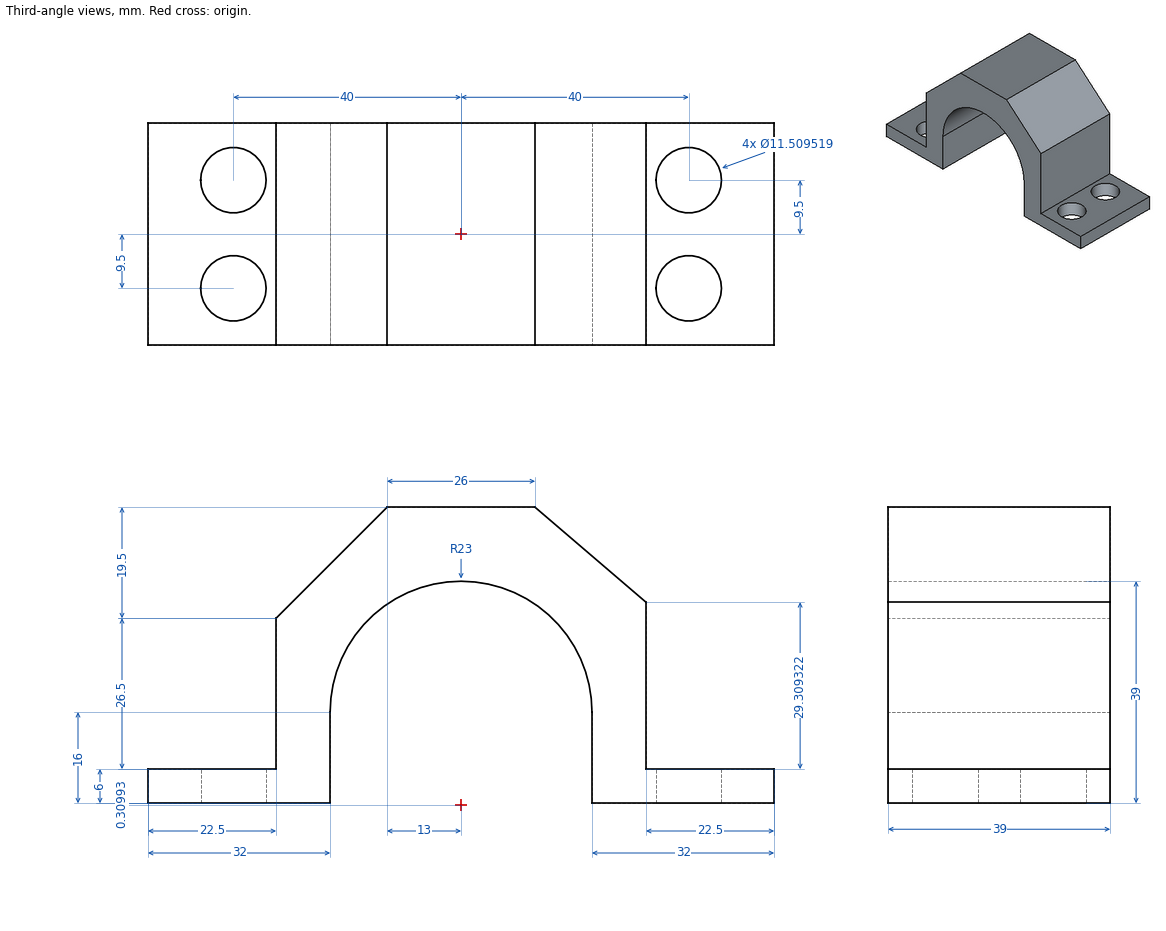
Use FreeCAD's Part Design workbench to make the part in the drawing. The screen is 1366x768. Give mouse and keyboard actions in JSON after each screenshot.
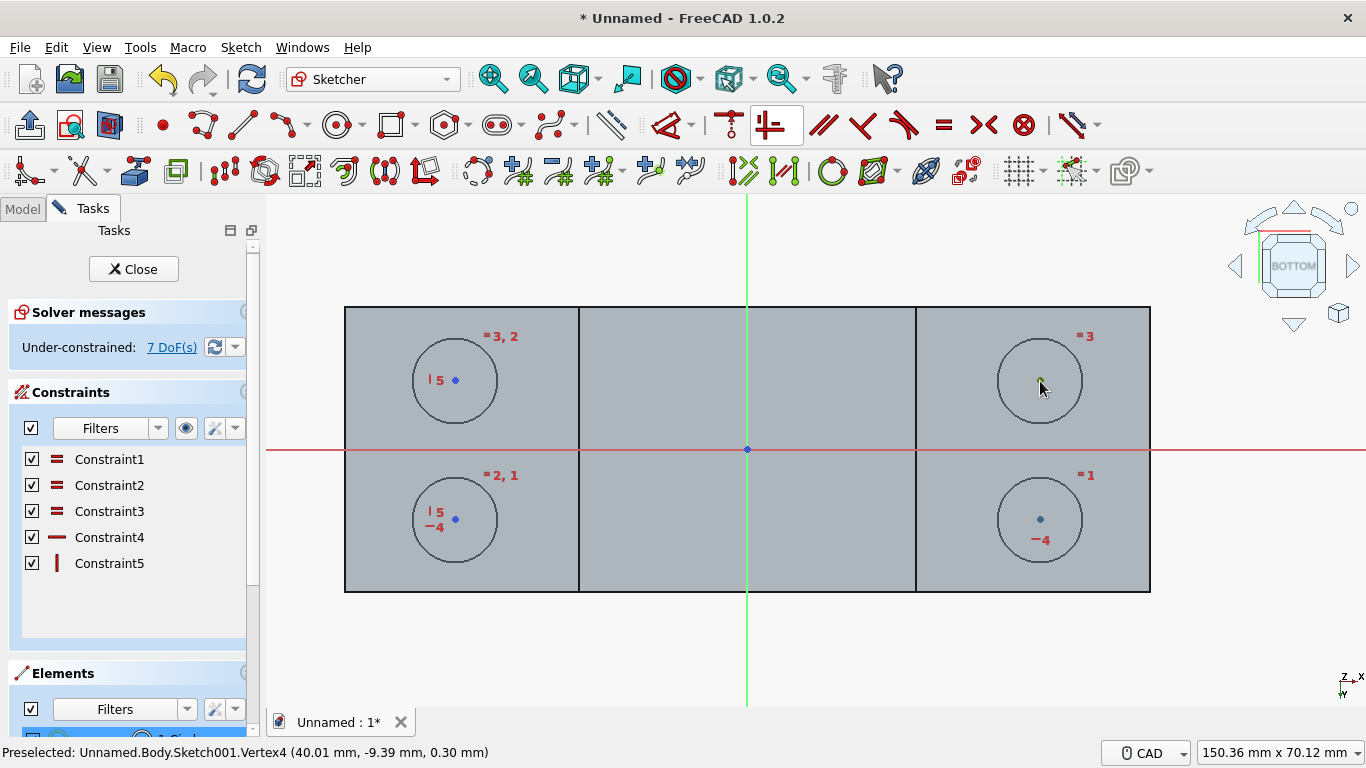
{"action": "key", "text": "v"}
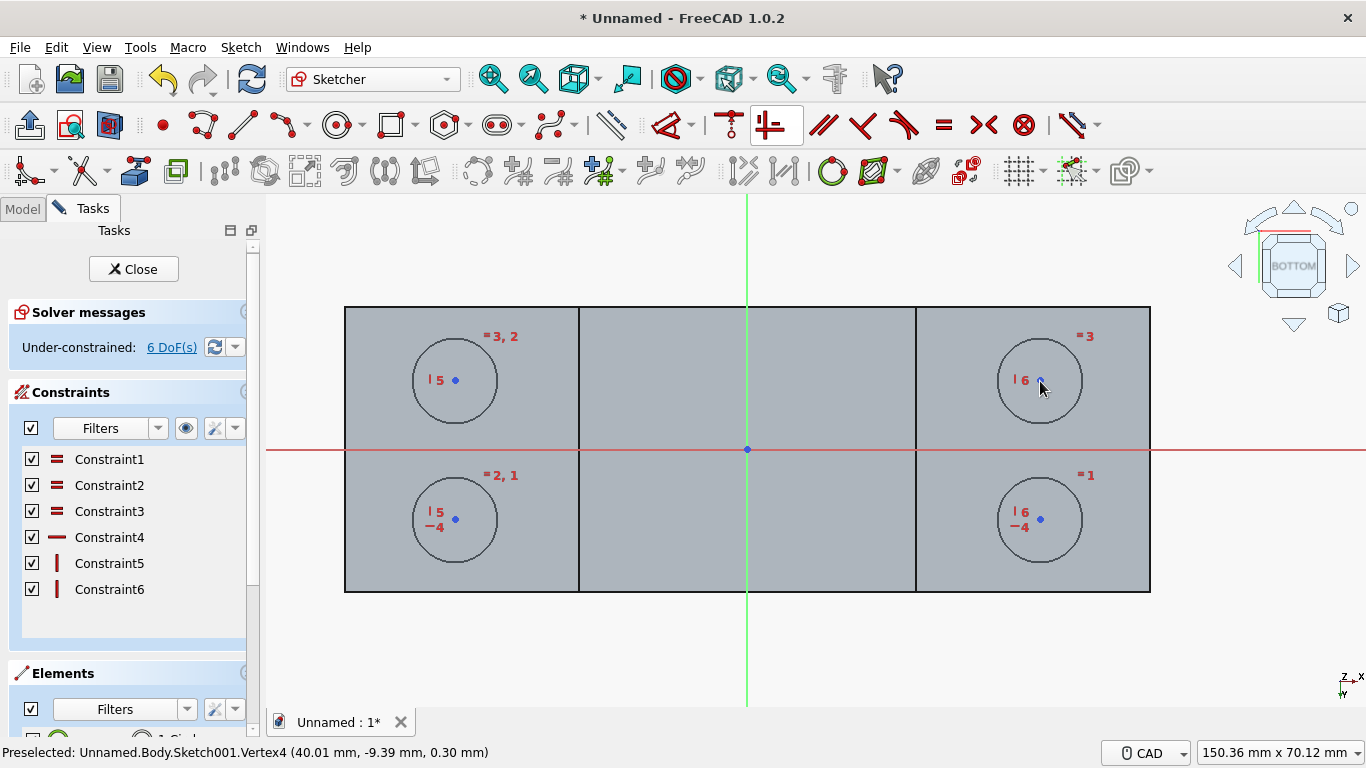
{"action": "left_click", "coordinate": [455, 381]}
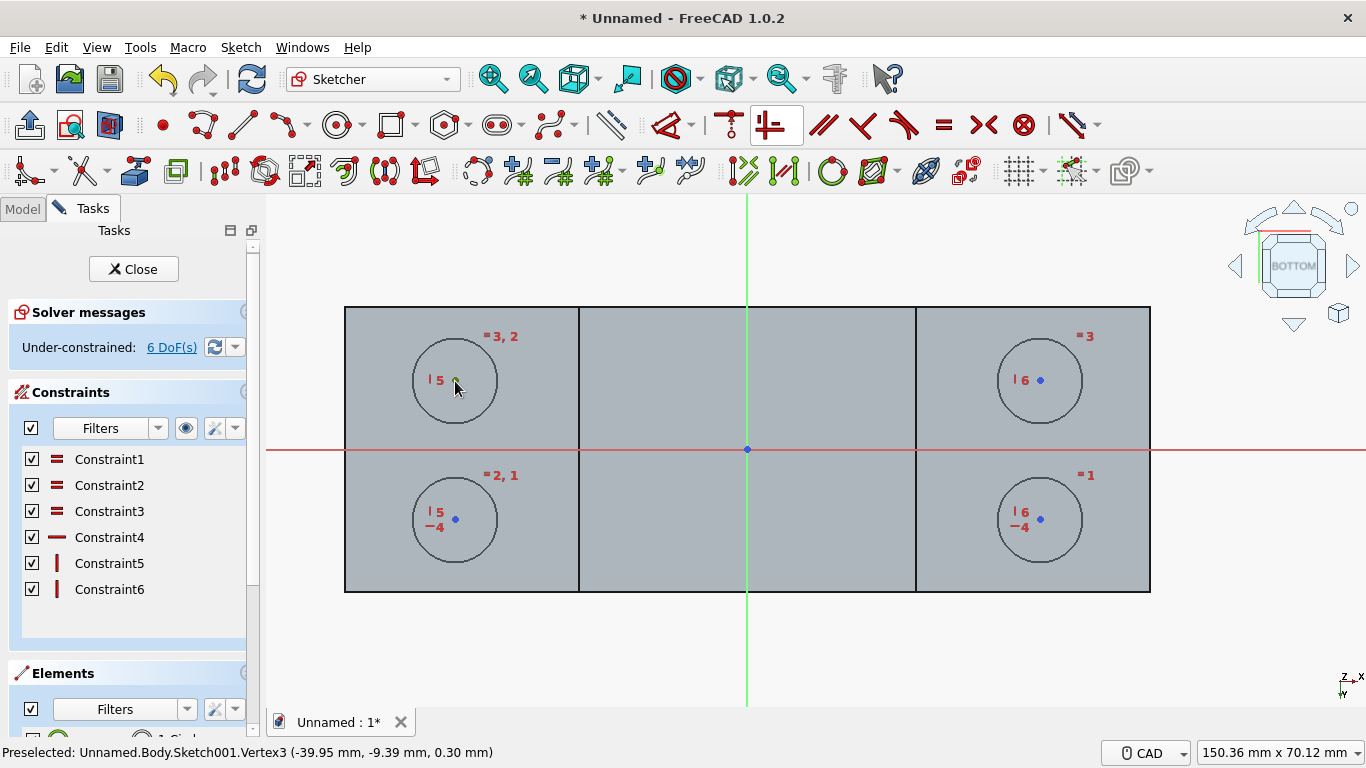
{"action": "left_click", "coordinate": [1040, 381]}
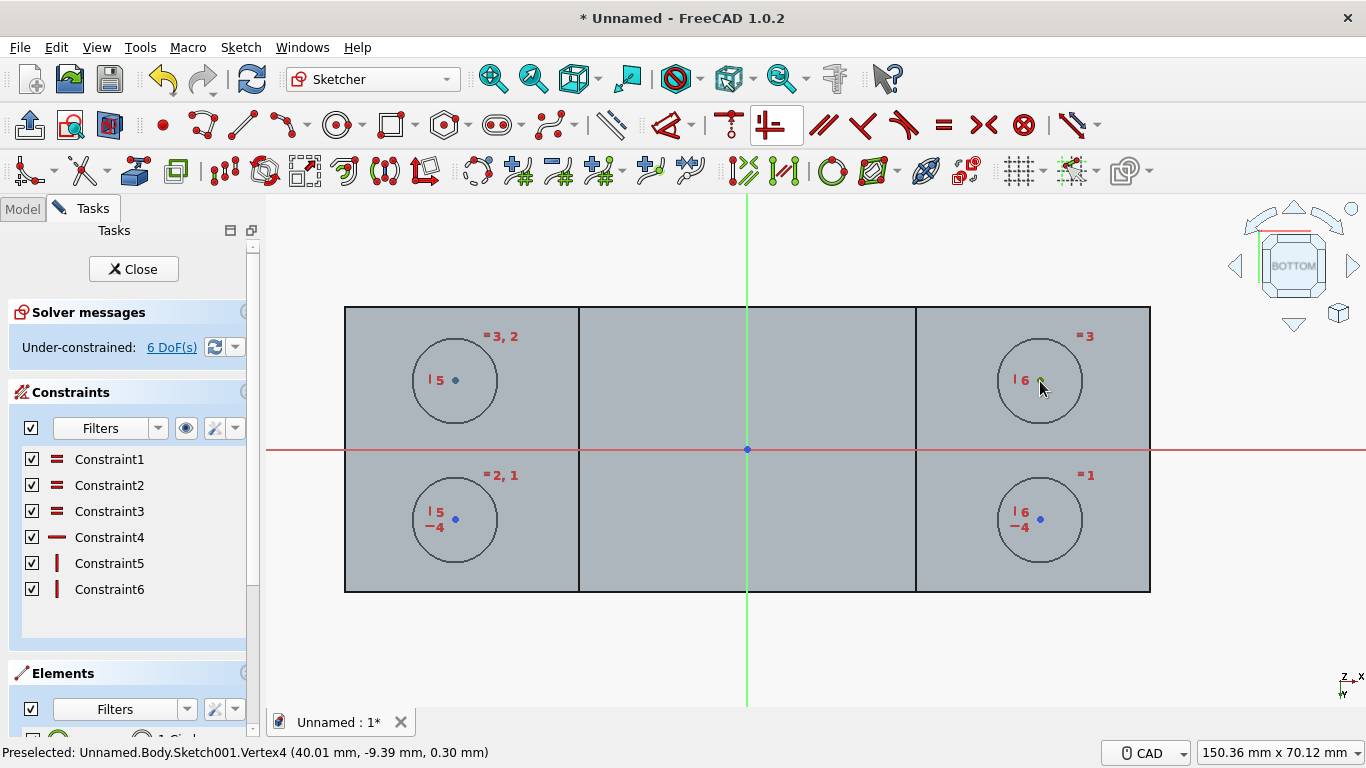
{"action": "key", "text": "h"}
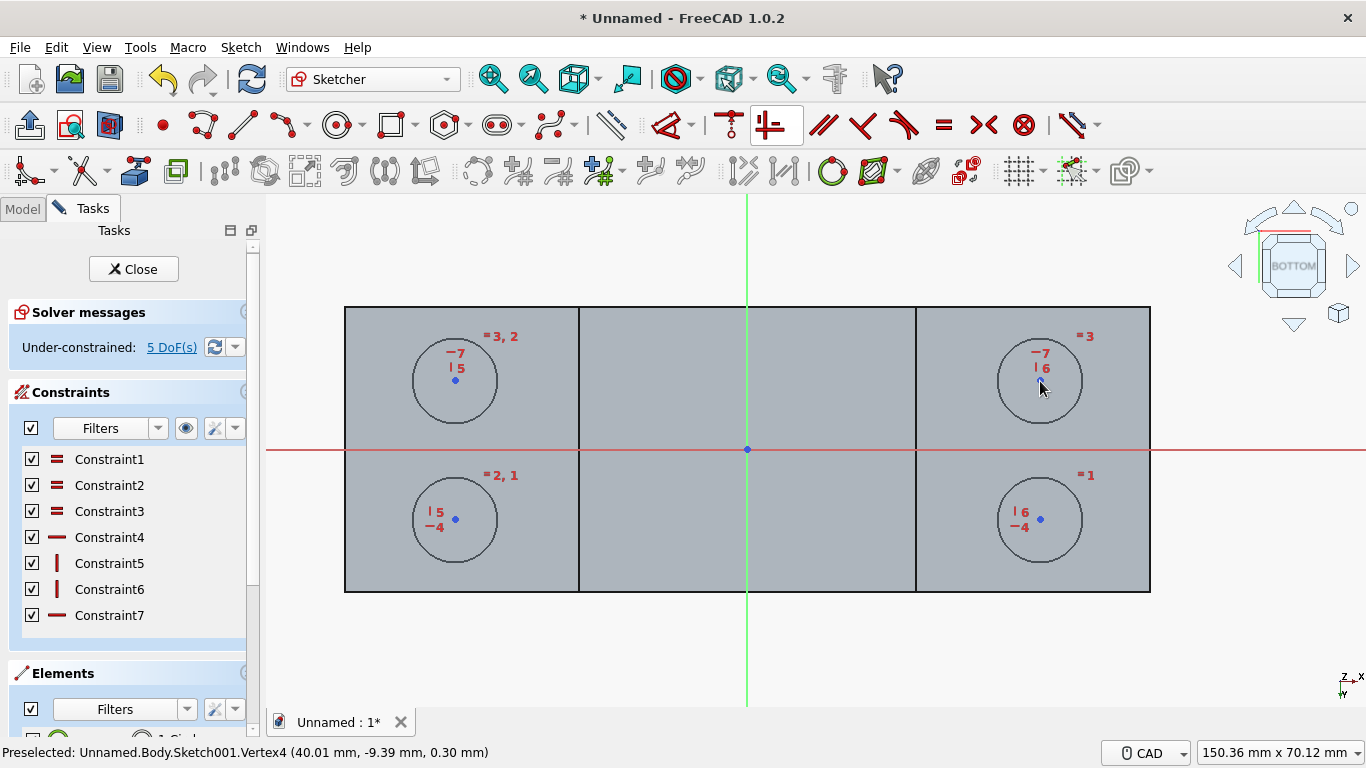
{"action": "left_click", "coordinate": [666, 126]}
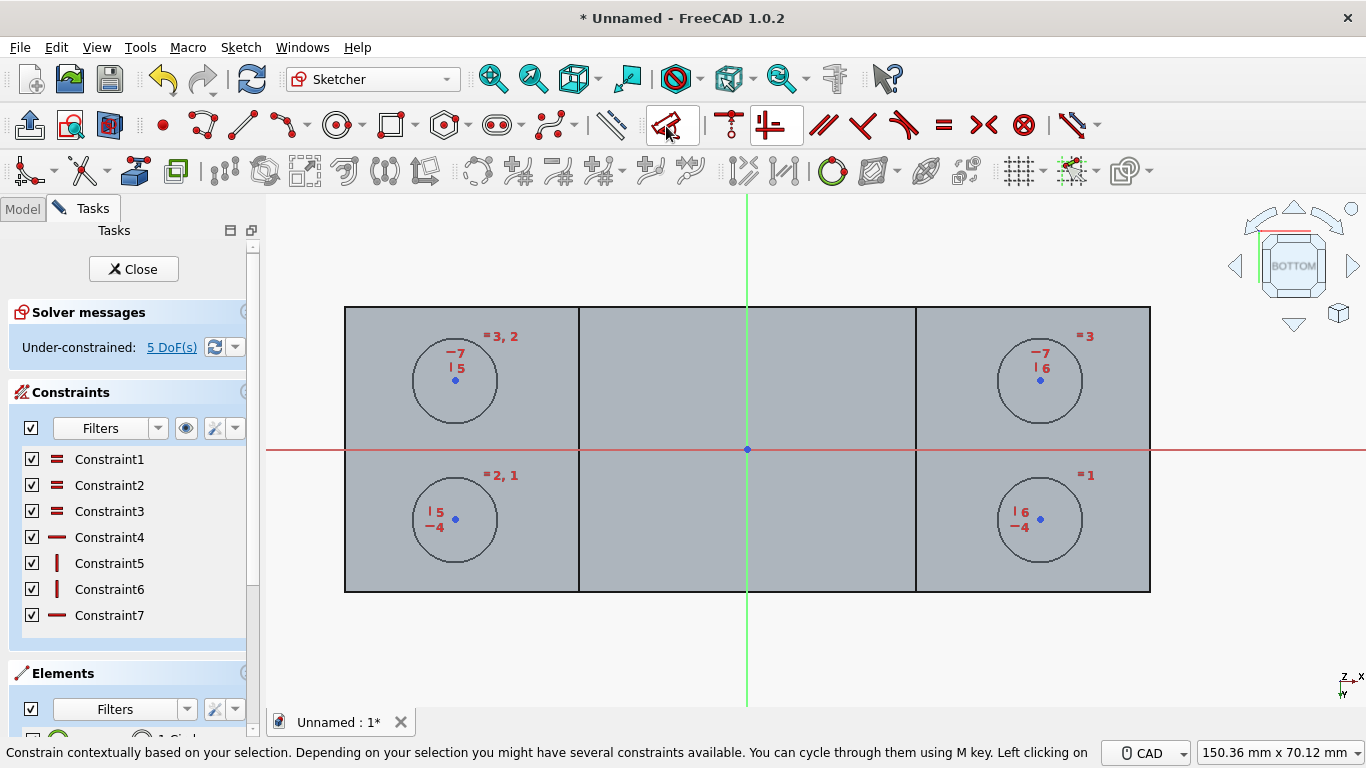
{"action": "left_click", "coordinate": [1070, 490]}
{"action": "left_click", "coordinate": [1093, 467]}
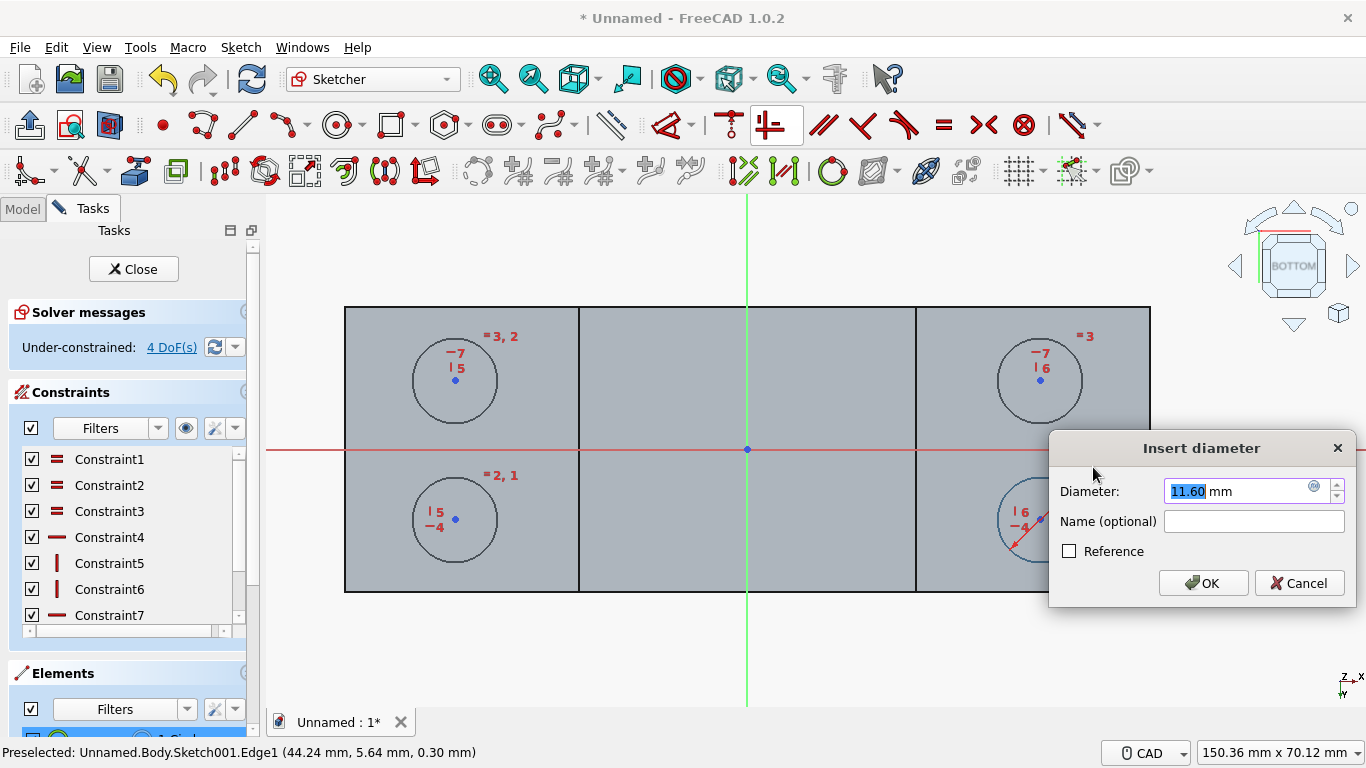
{"action": "type", "text": "11.509519"}
{"action": "key", "text": "Return"}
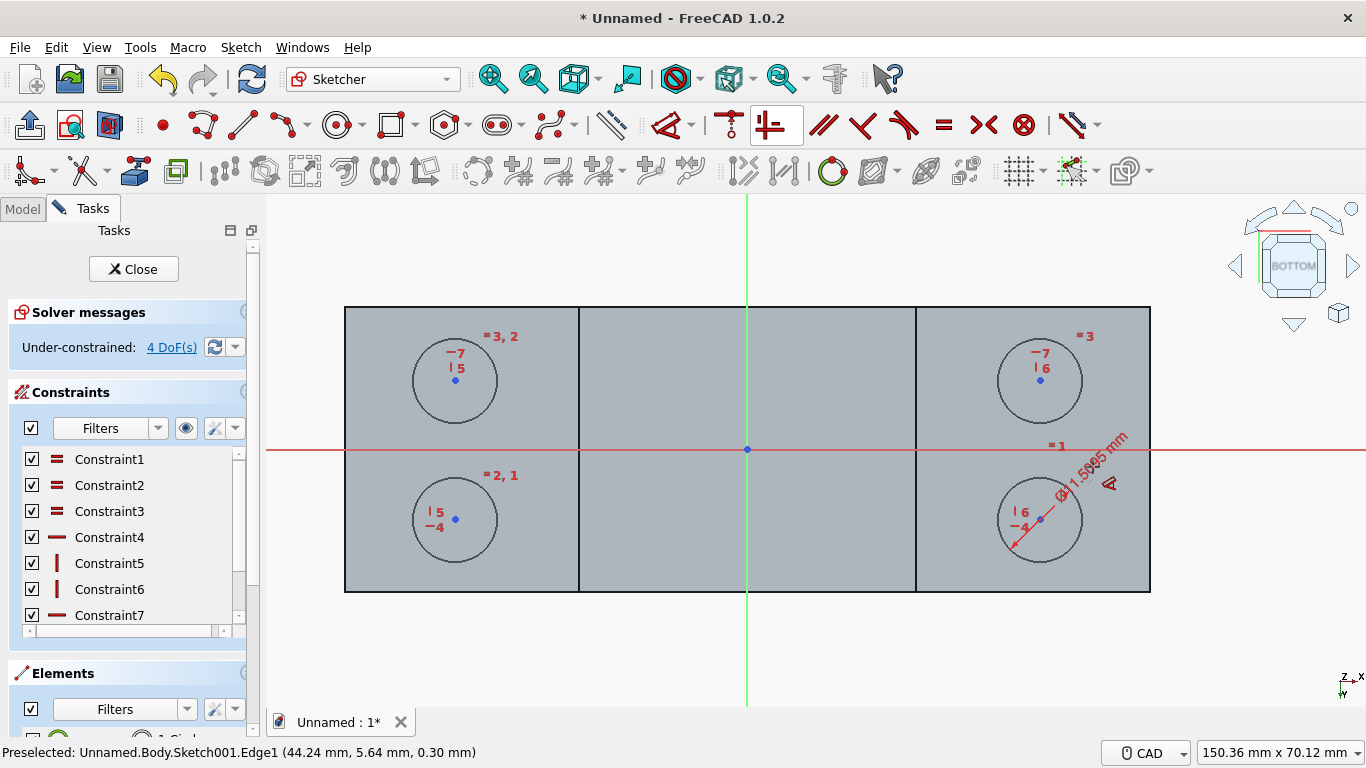
{"action": "left_click", "coordinate": [1040, 520]}
{"action": "left_click", "coordinate": [894, 554]}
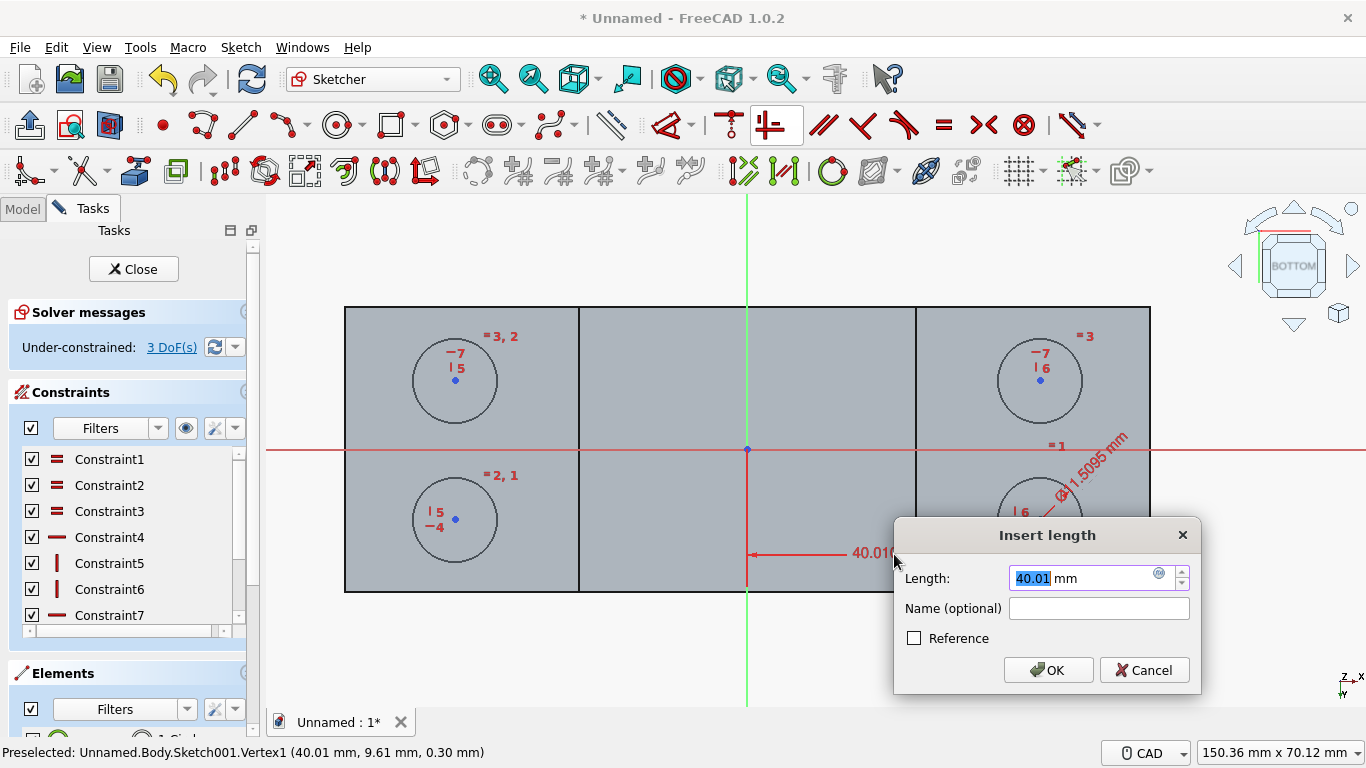
{"action": "type", "text": "40"}
{"action": "key", "text": "Return"}